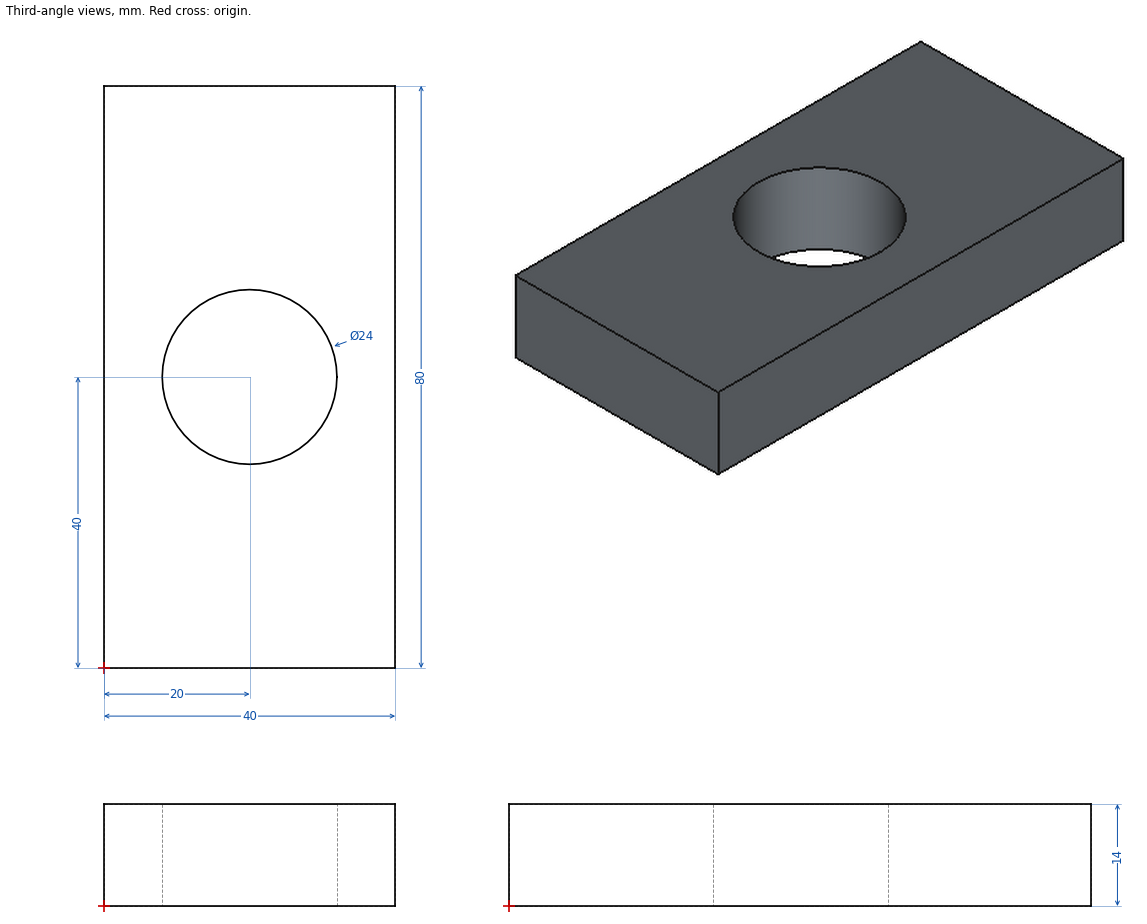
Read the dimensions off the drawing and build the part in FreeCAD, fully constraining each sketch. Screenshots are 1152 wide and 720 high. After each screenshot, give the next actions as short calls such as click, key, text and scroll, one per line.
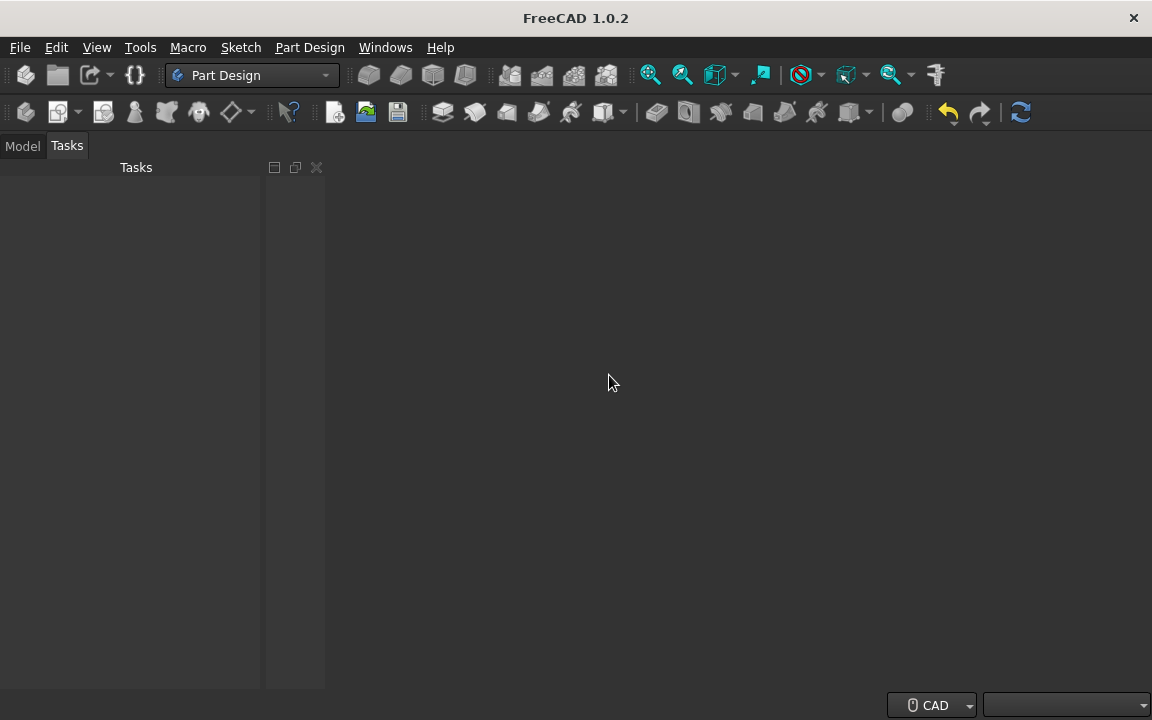
click(334, 112)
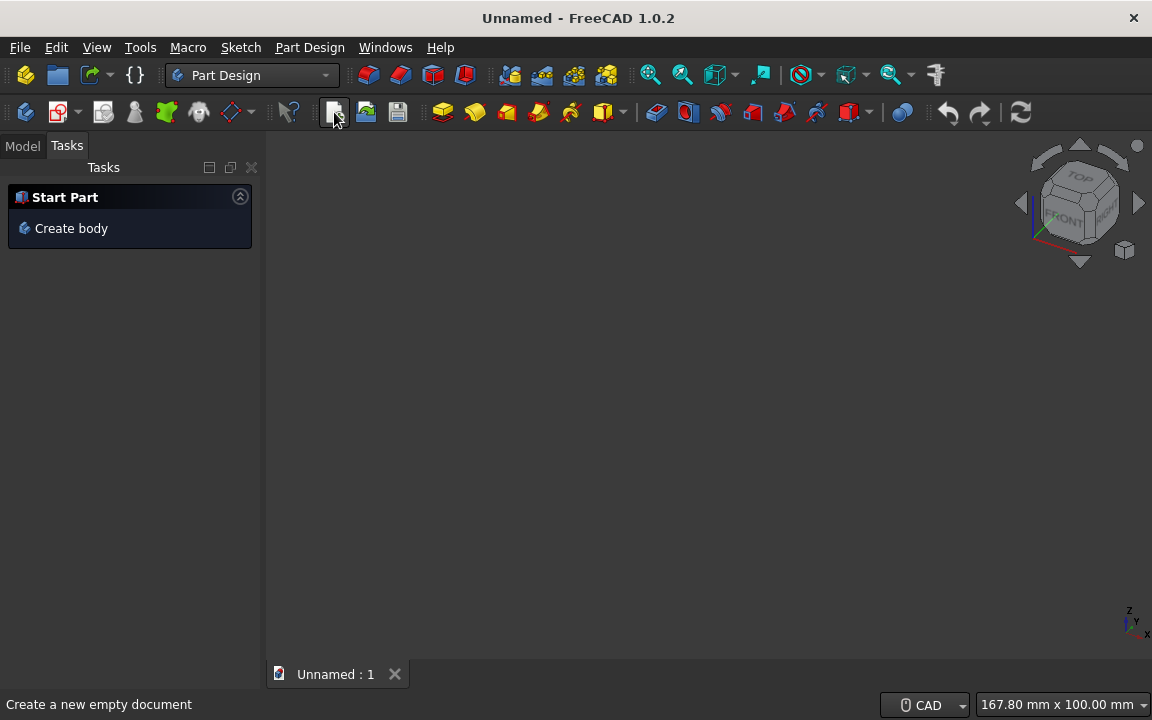
click(58, 112)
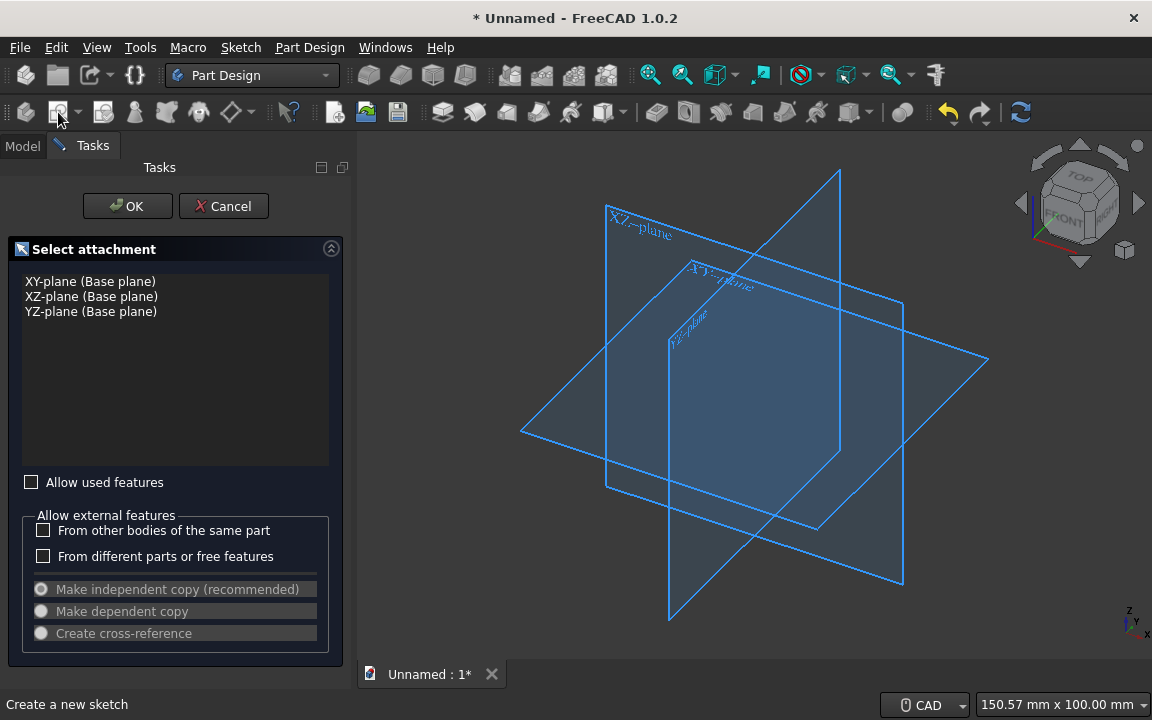
click(82, 282)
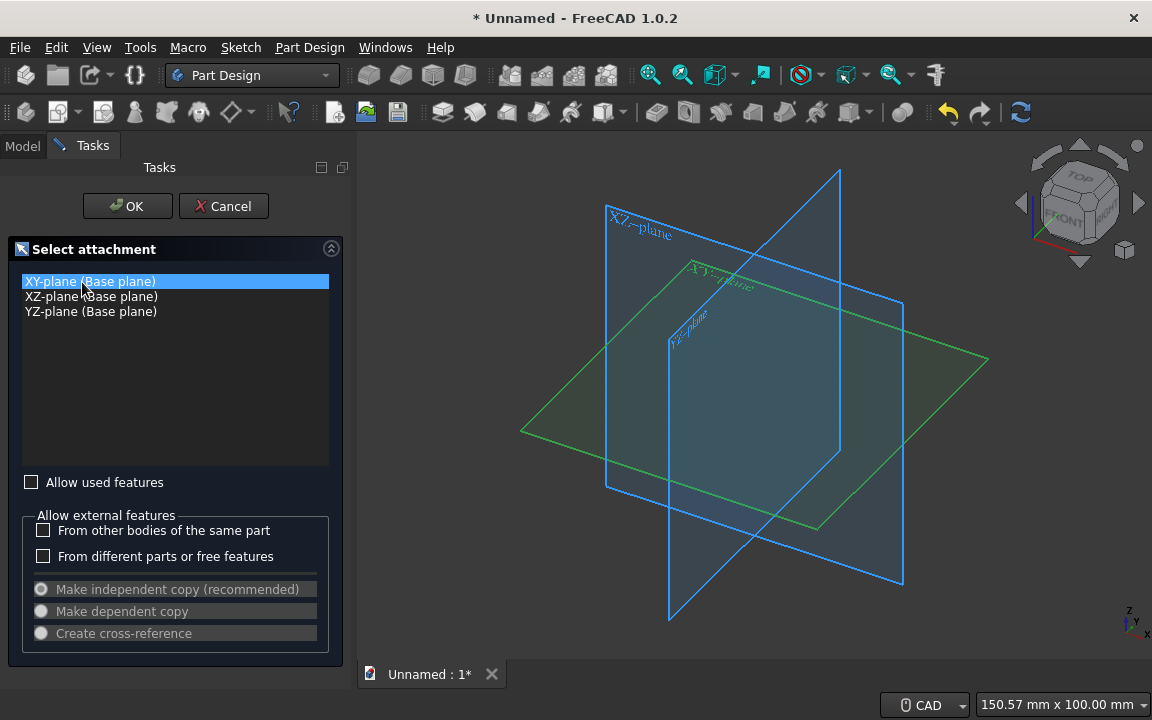
click(128, 206)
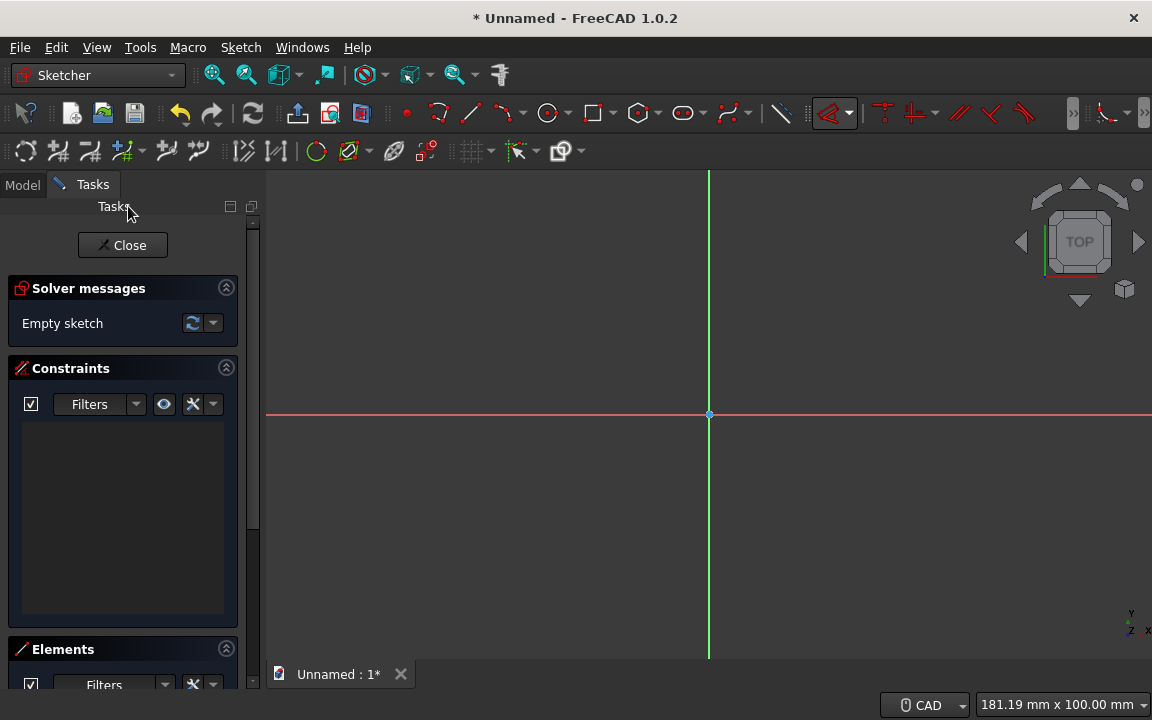
scroll(302, 631, down, 2)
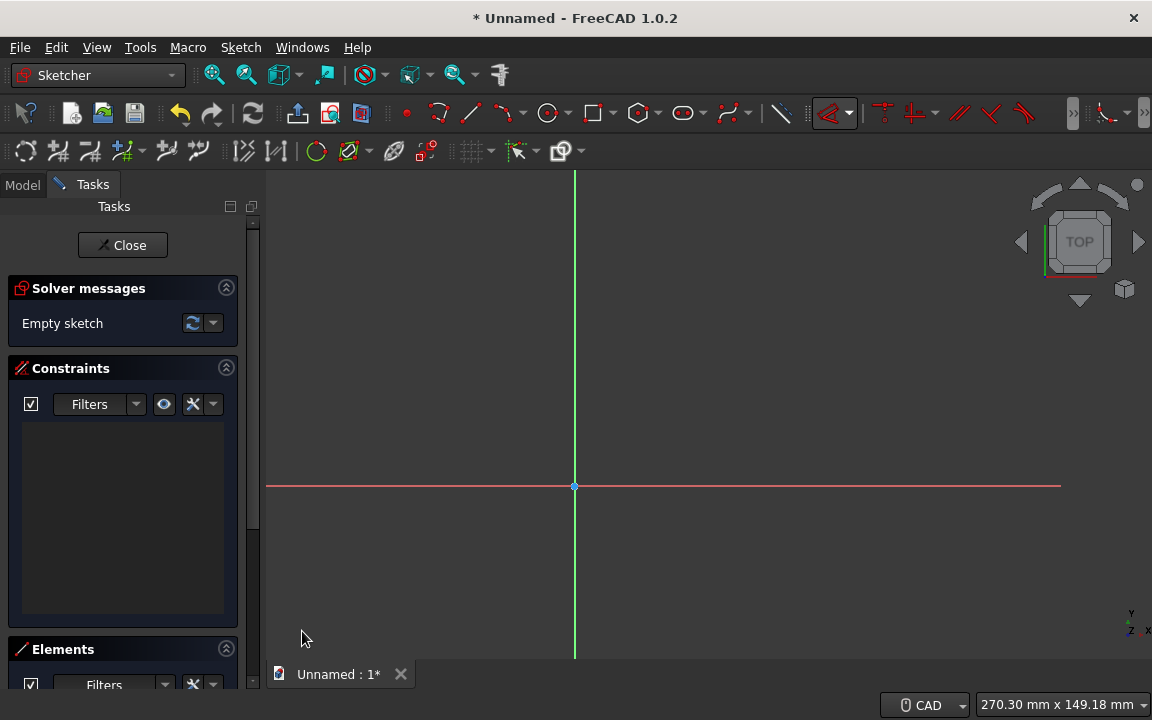
click(594, 114)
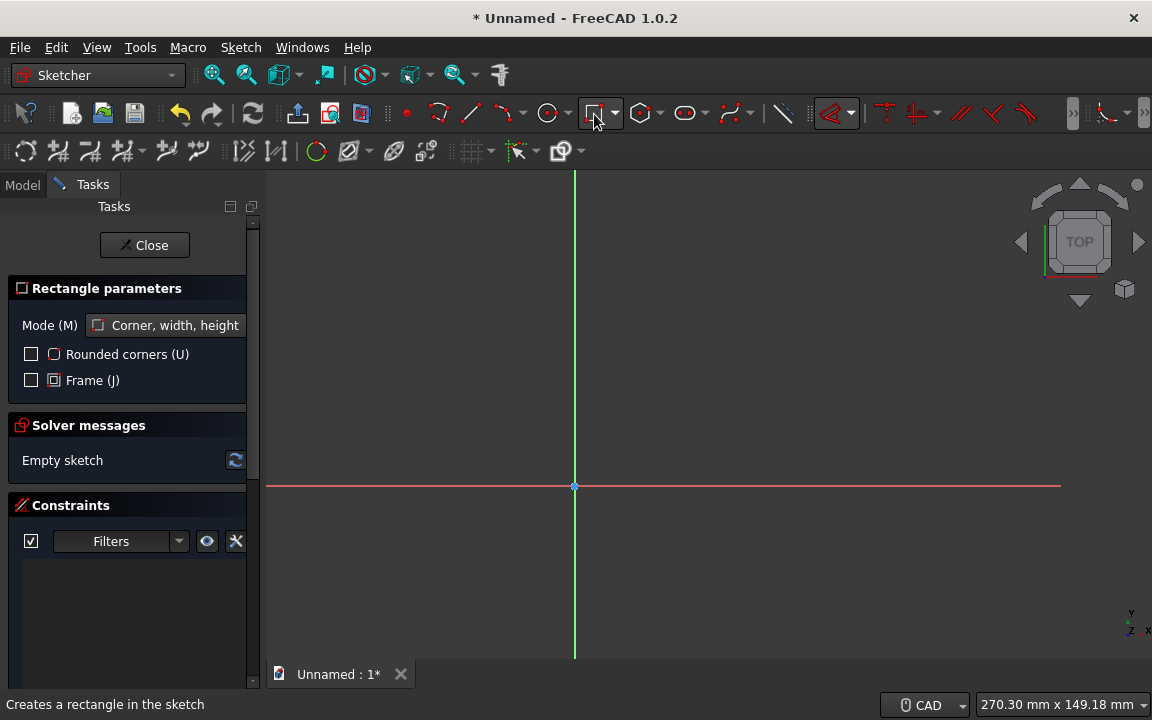
click(575, 486)
move(706, 224)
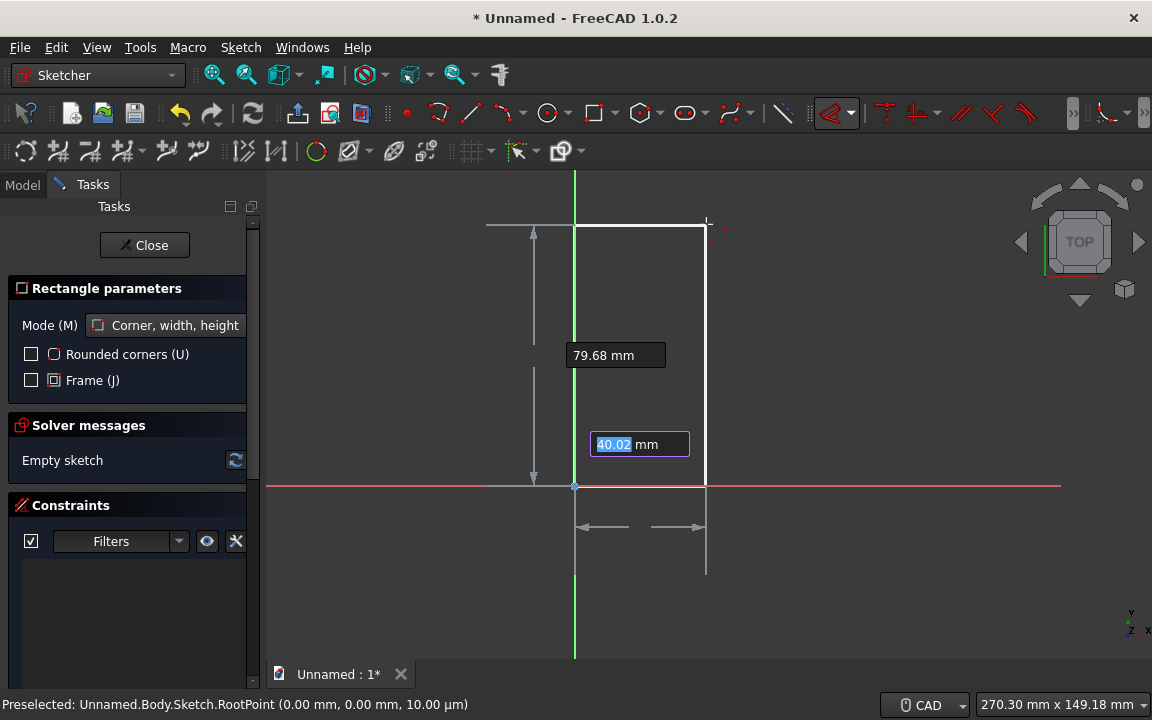
text(40)
key(Tab)
text(80)
key(Return)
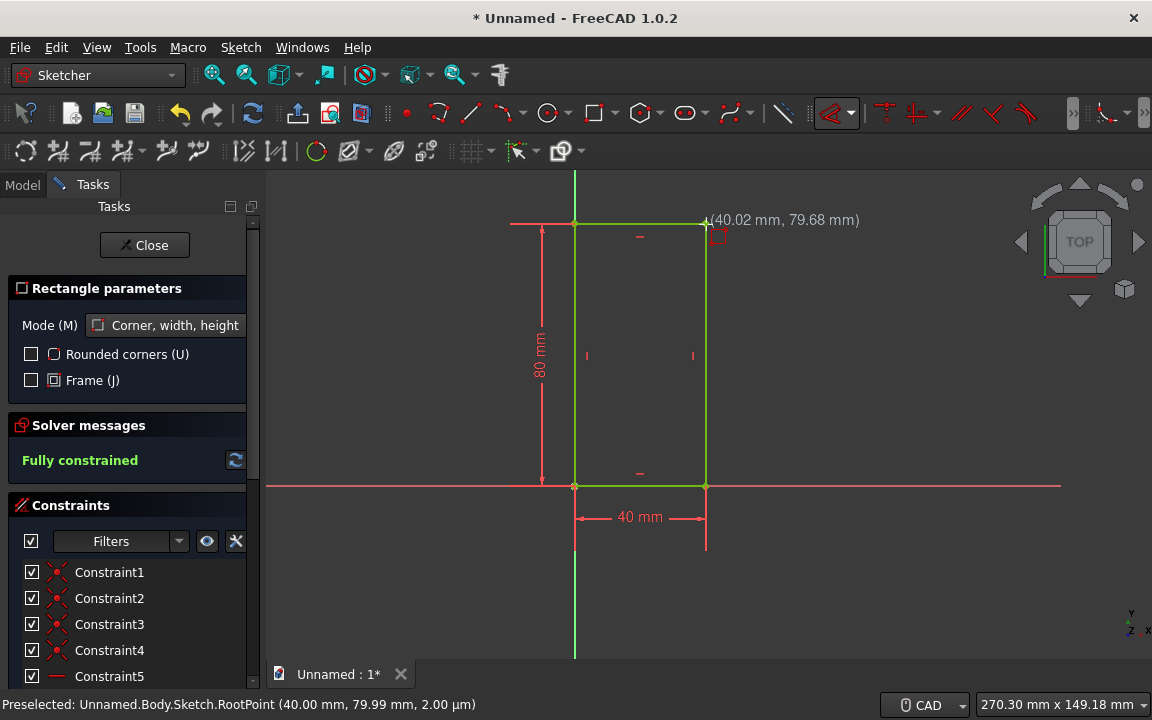
click(548, 114)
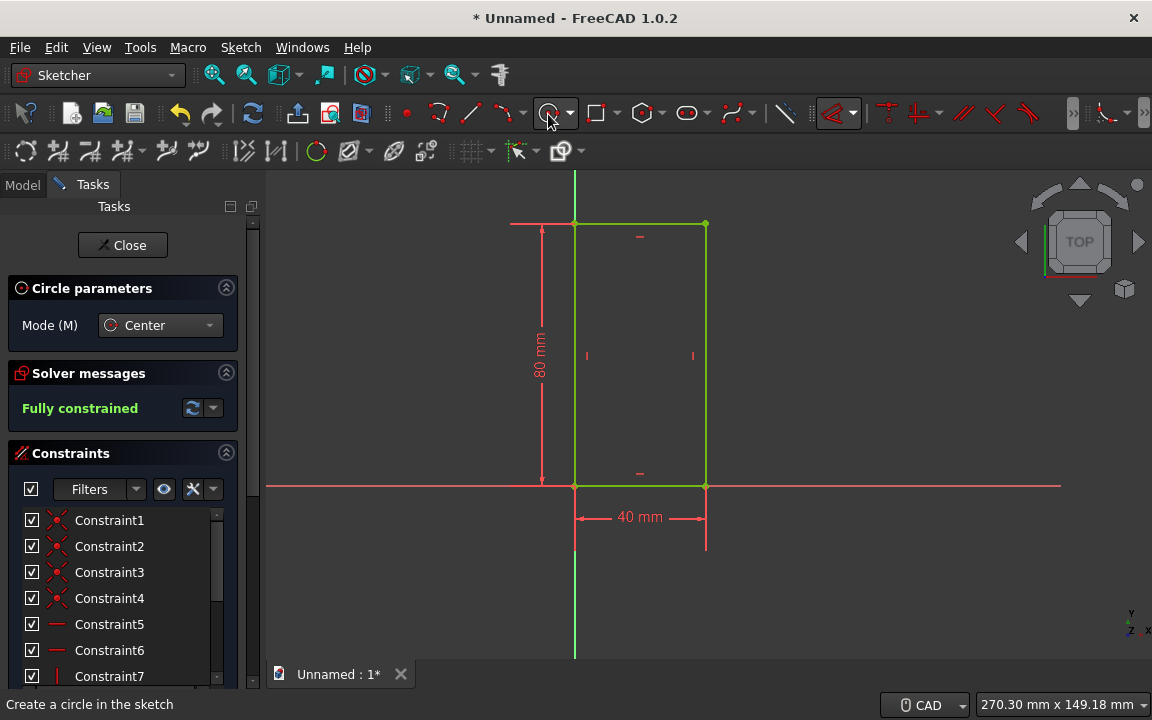
click(640, 355)
move(668, 327)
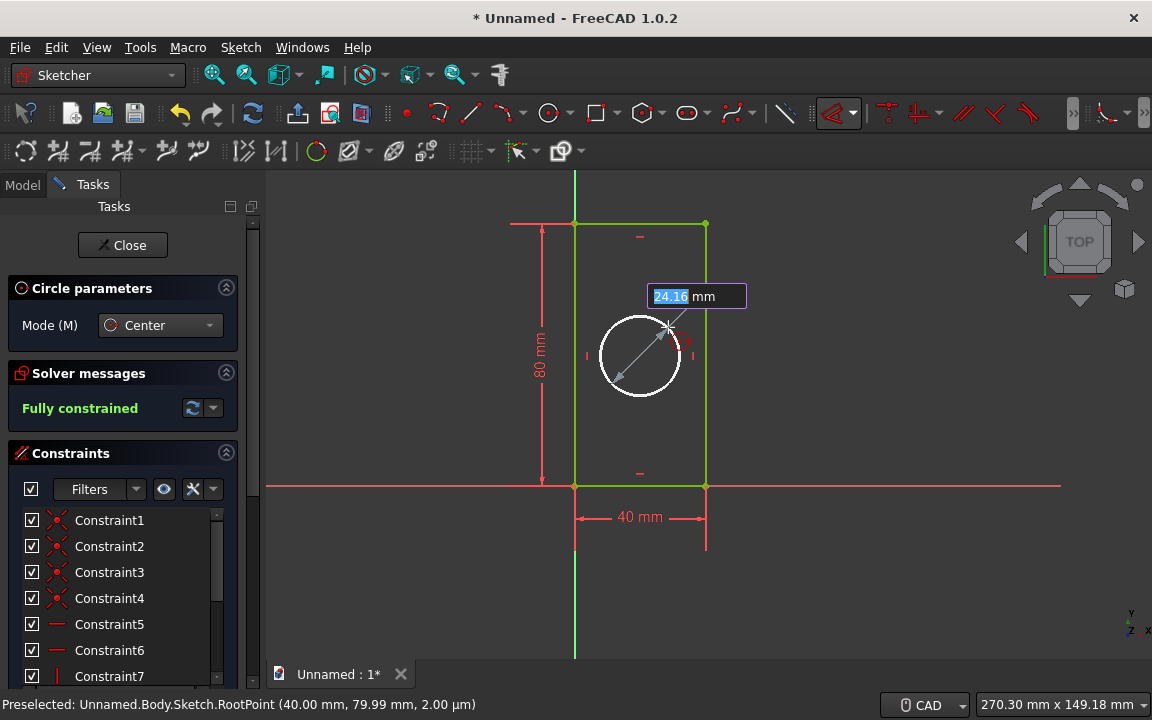
text(24)
key(Return)
key(Escape)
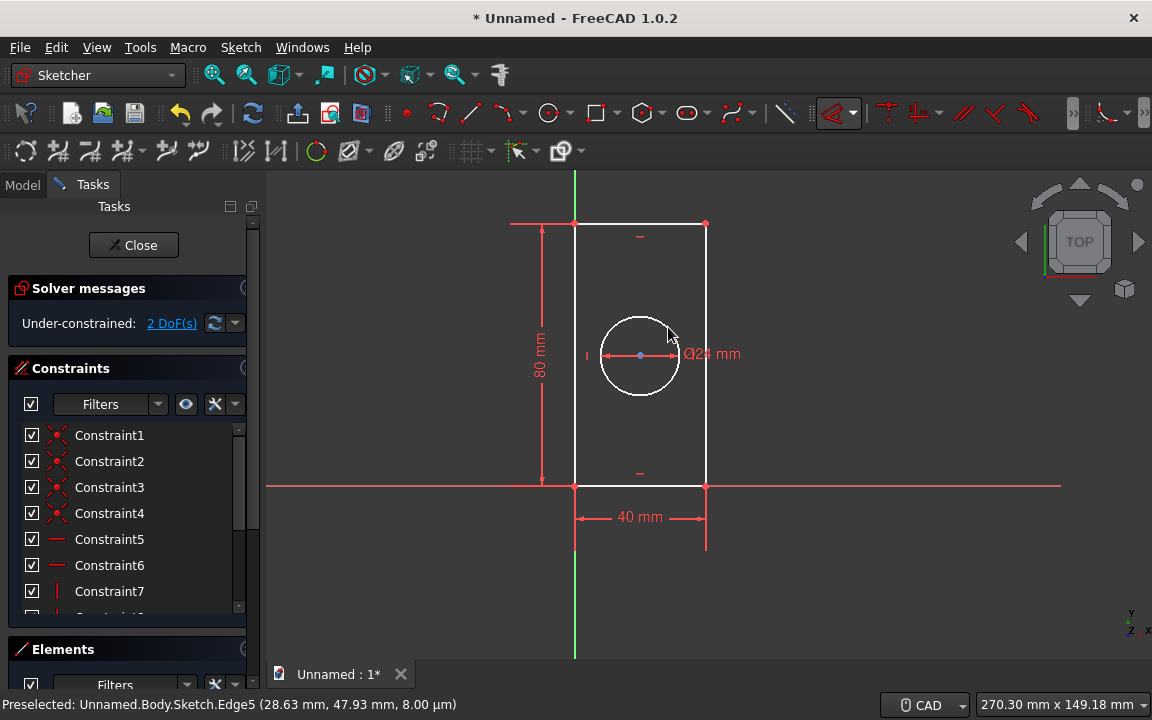
click(832, 114)